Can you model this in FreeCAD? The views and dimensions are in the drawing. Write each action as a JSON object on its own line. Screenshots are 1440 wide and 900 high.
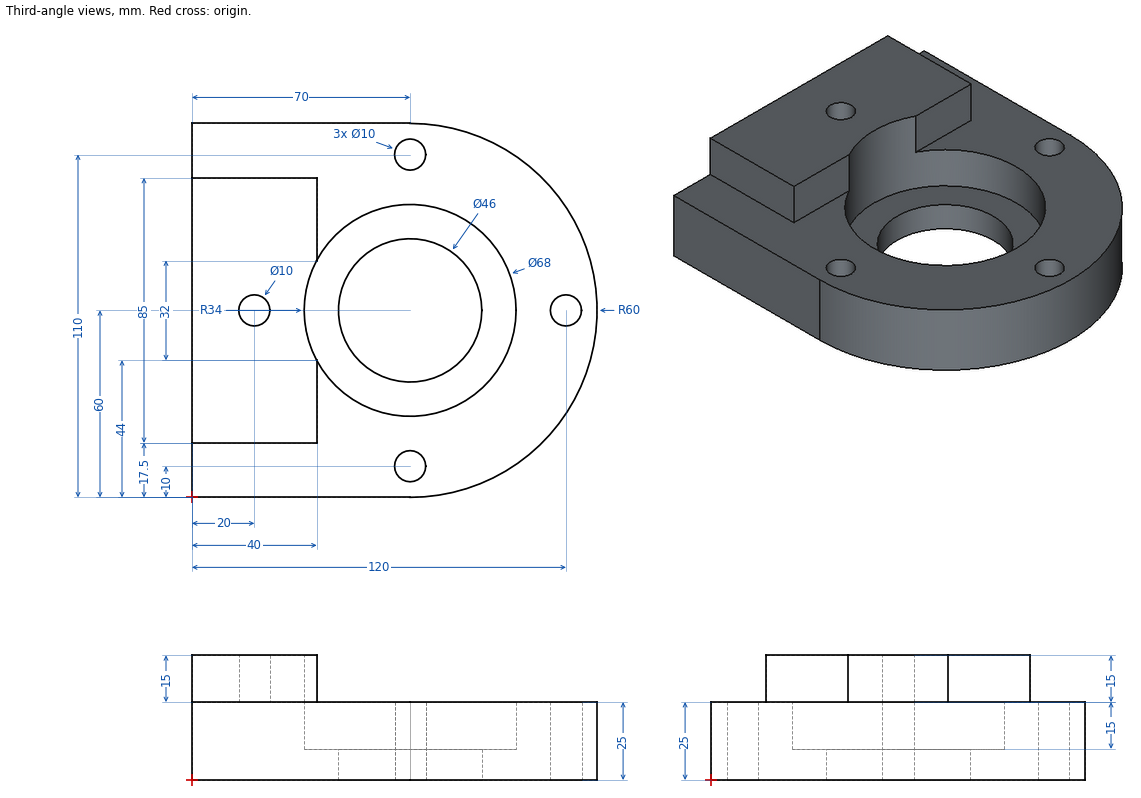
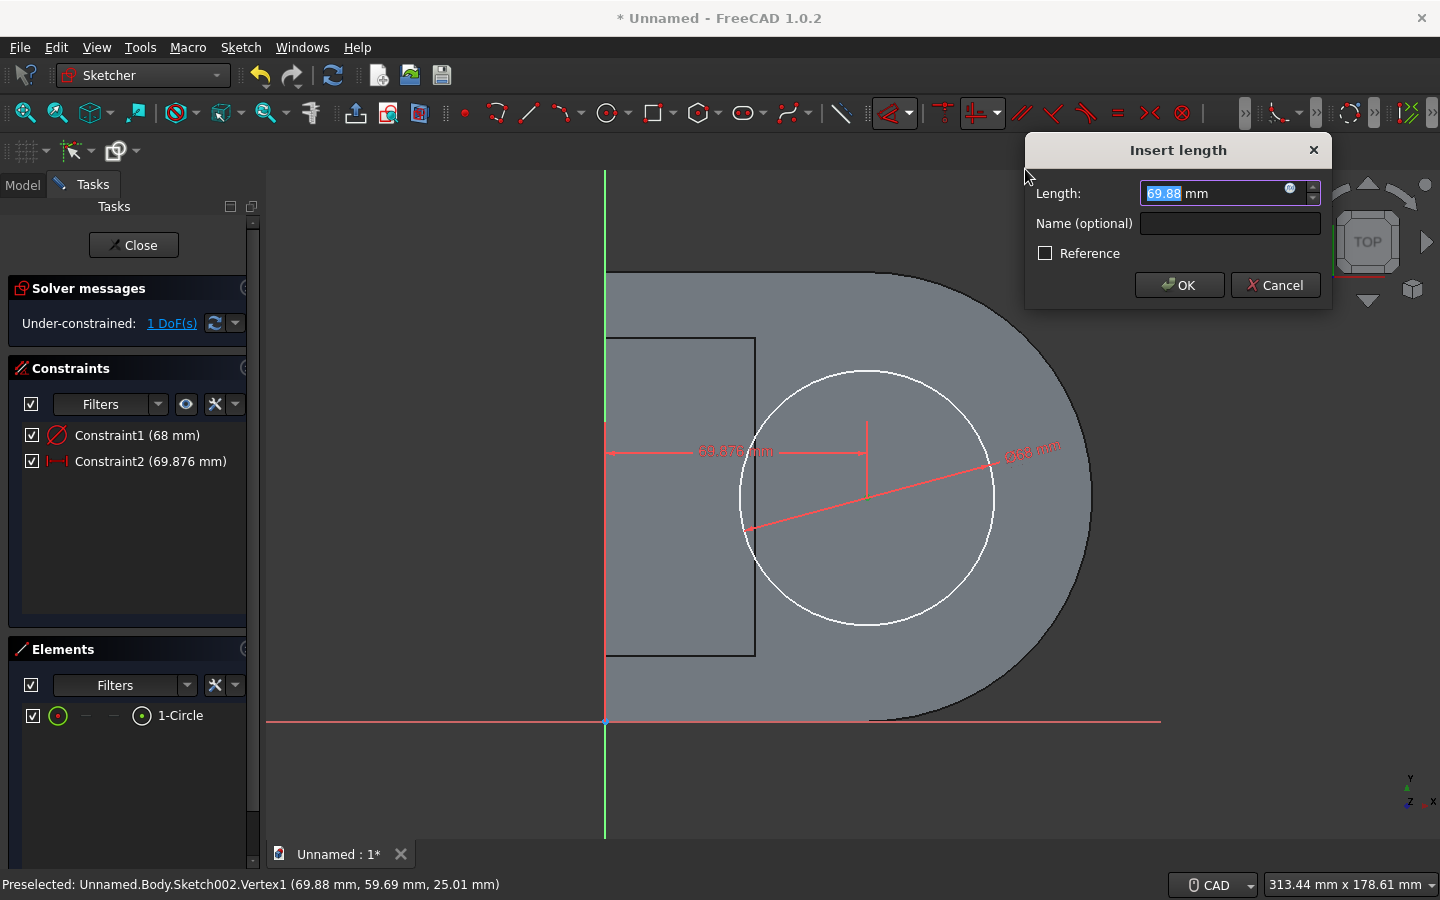
{"action": "type", "text": "70"}
{"action": "key", "text": "Return"}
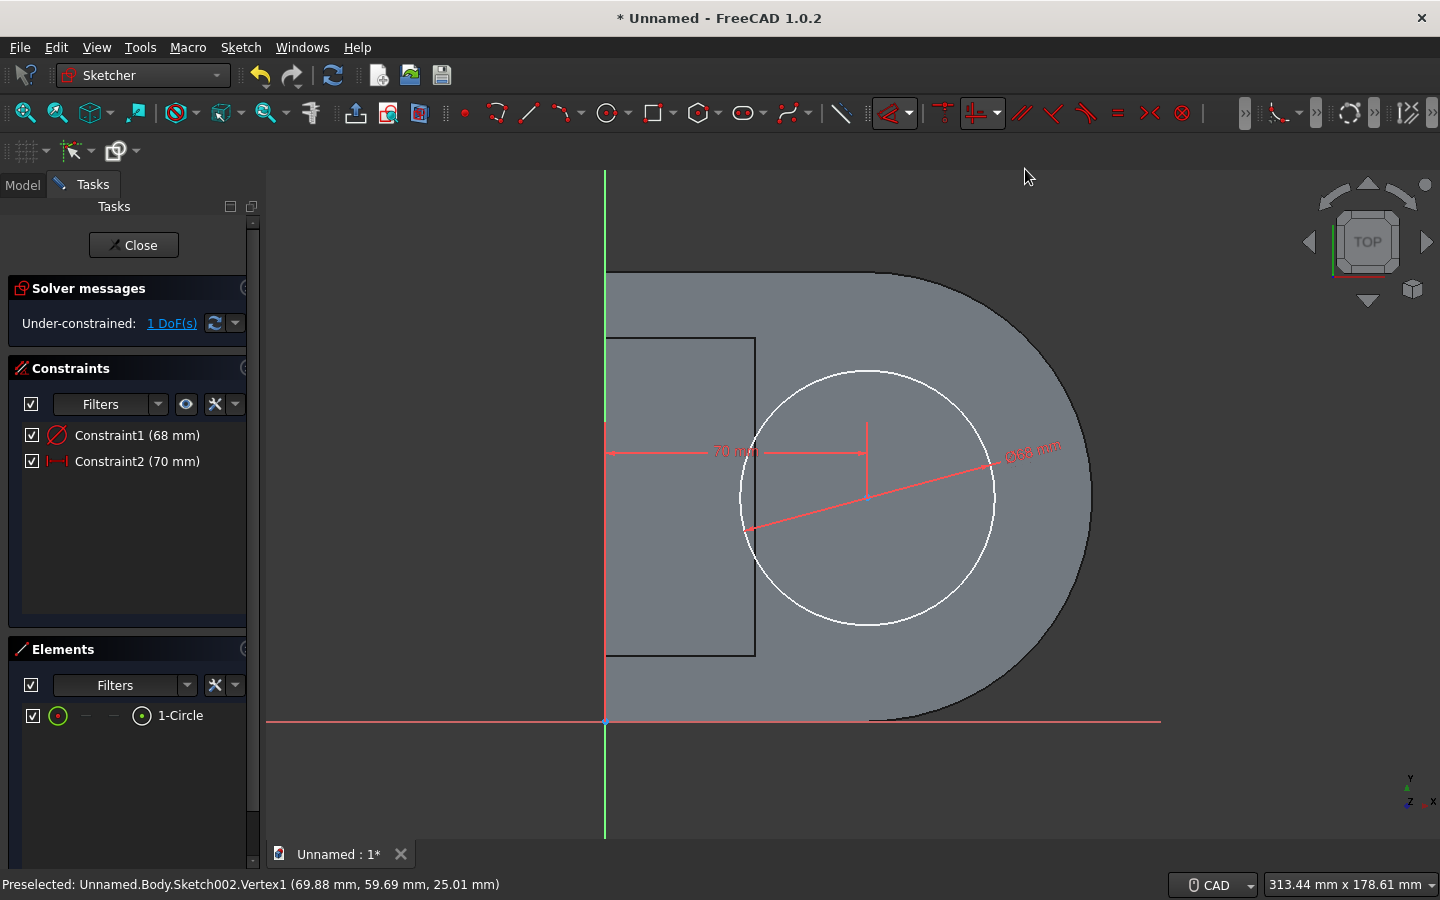
{"action": "left_click", "coordinate": [867, 498]}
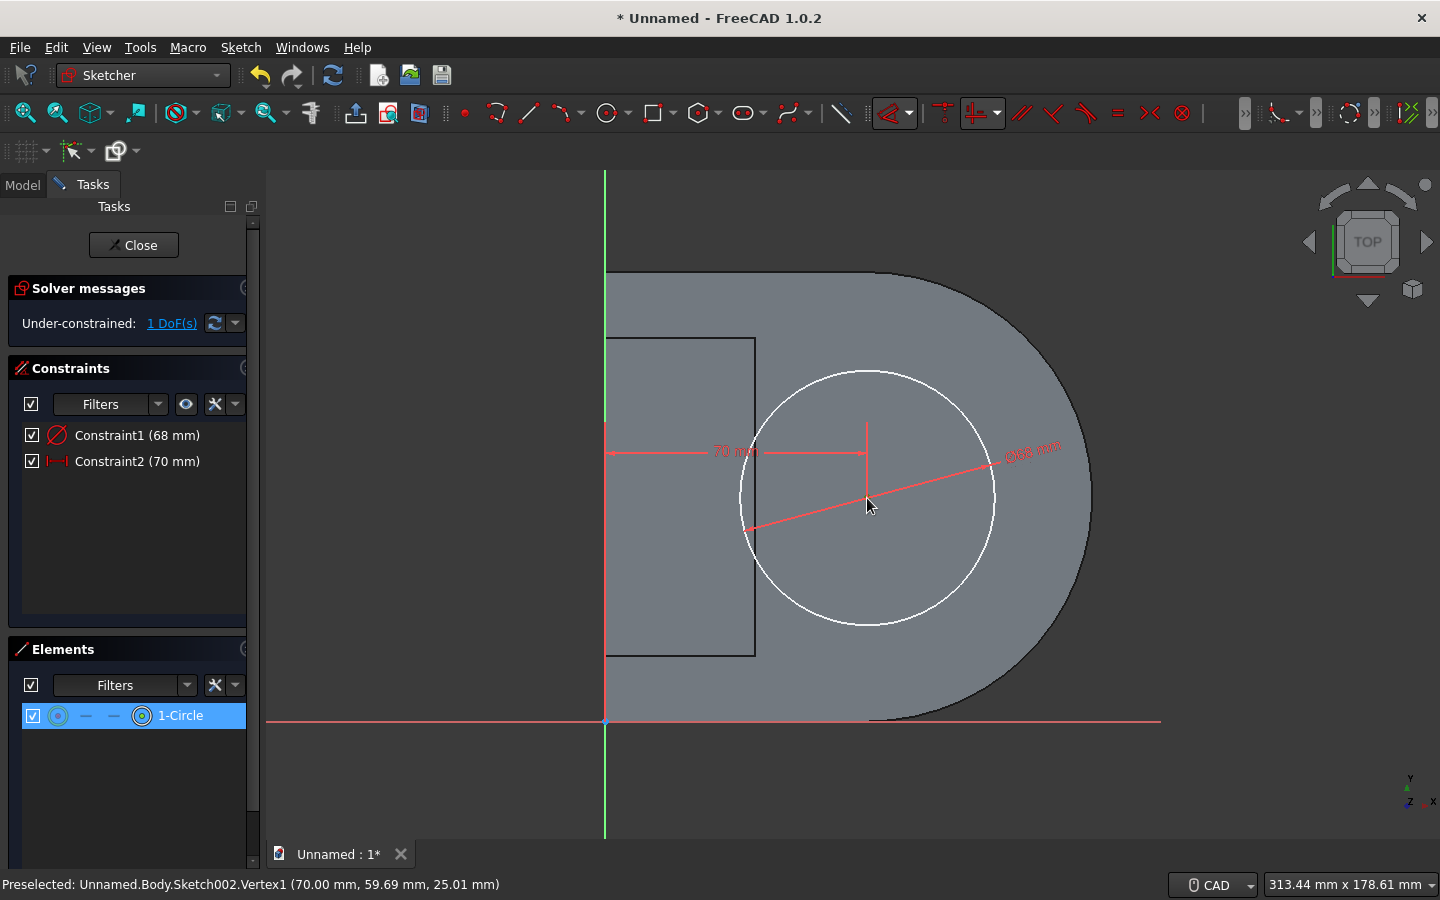
{"action": "left_click", "coordinate": [912, 114]}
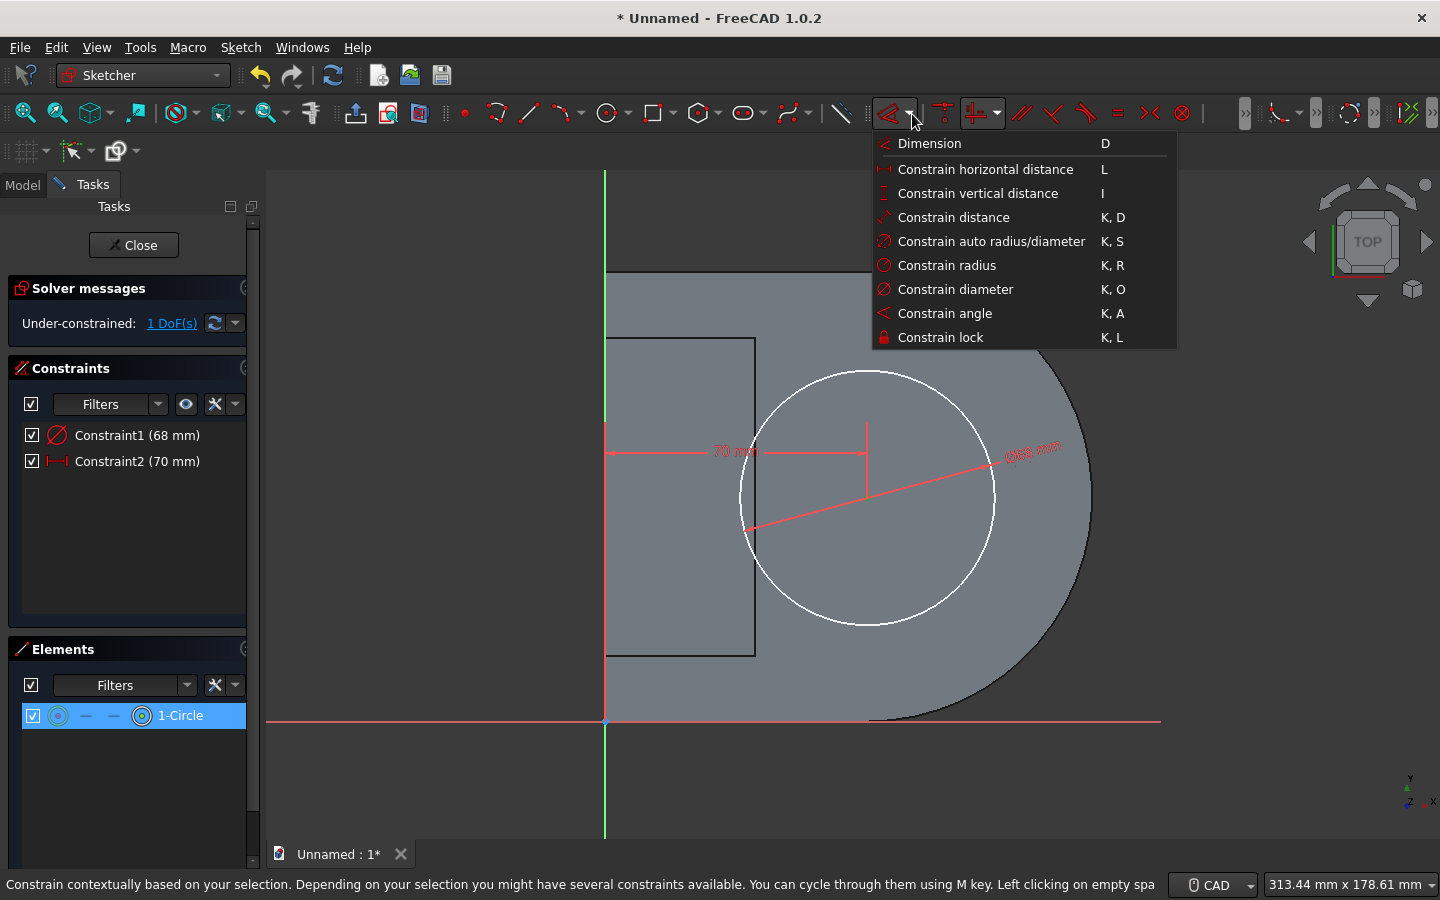
{"action": "left_click", "coordinate": [1025, 193]}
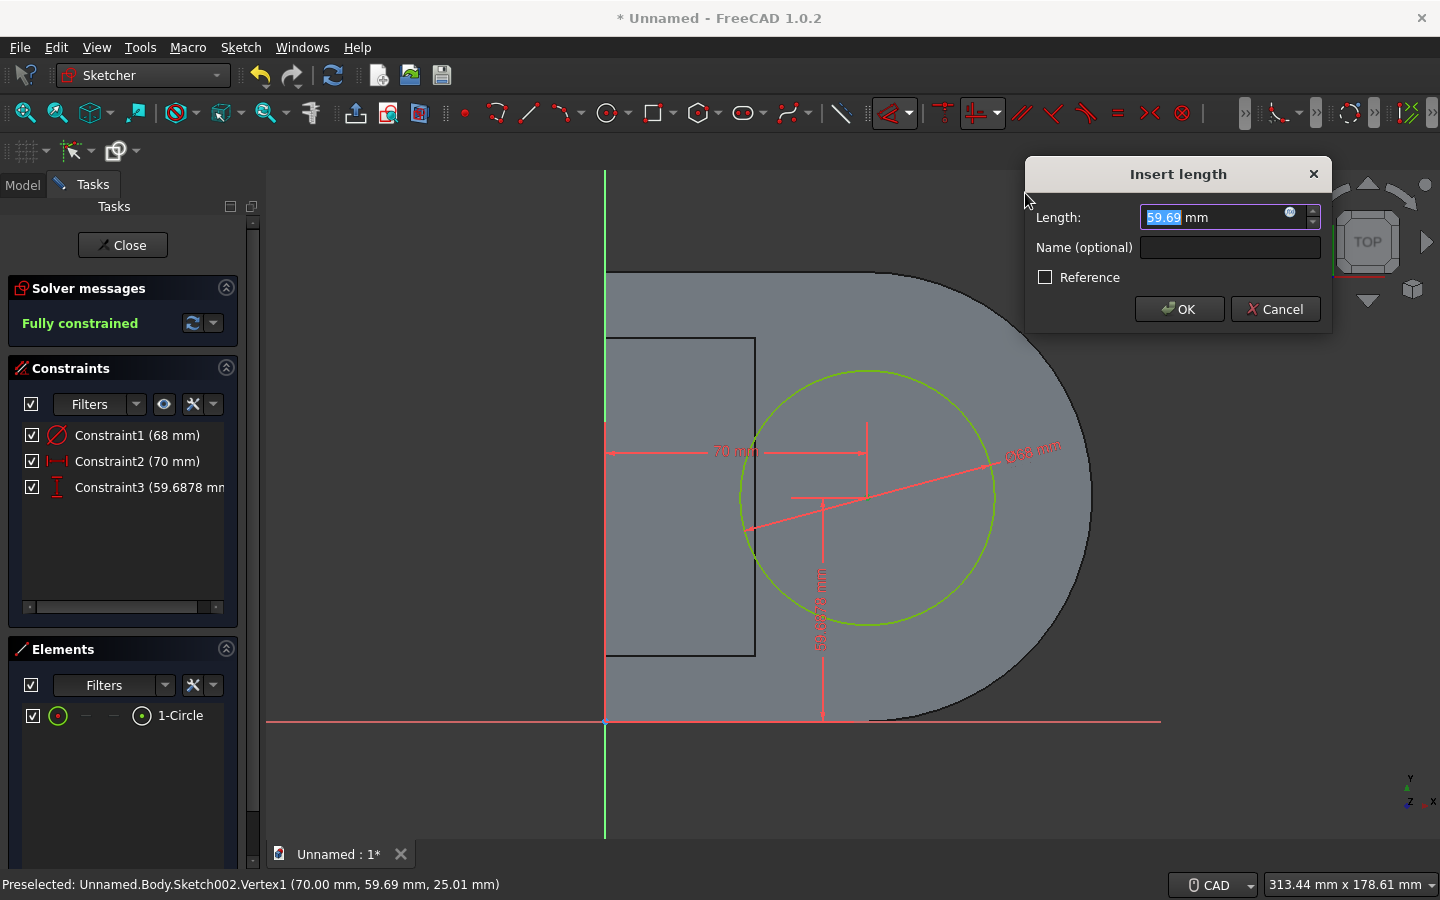
{"action": "type", "text": "60"}
{"action": "key", "text": "Return"}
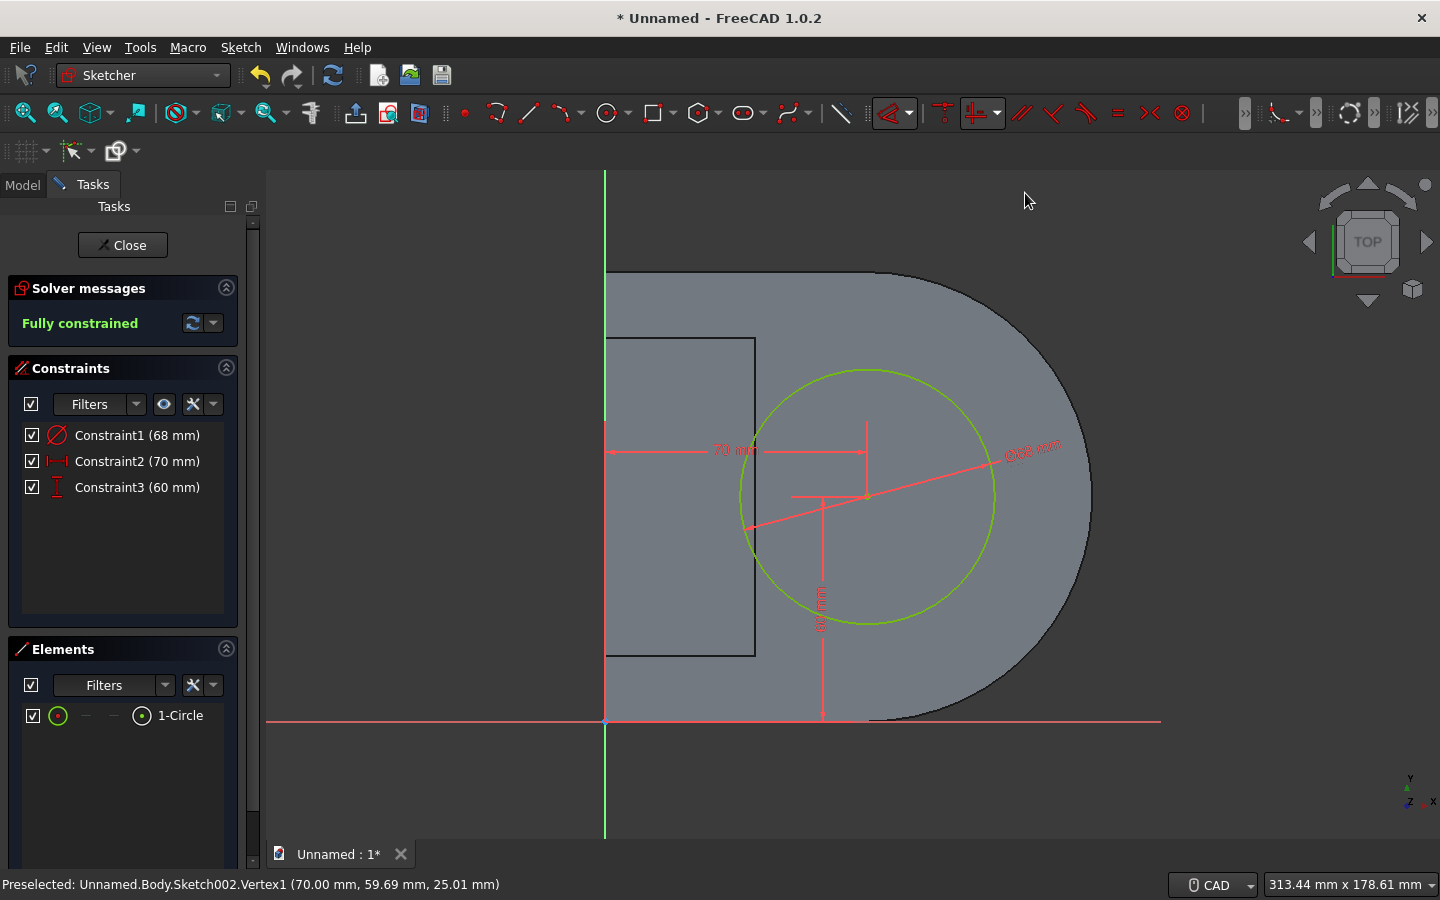
{"action": "left_click", "coordinate": [123, 245]}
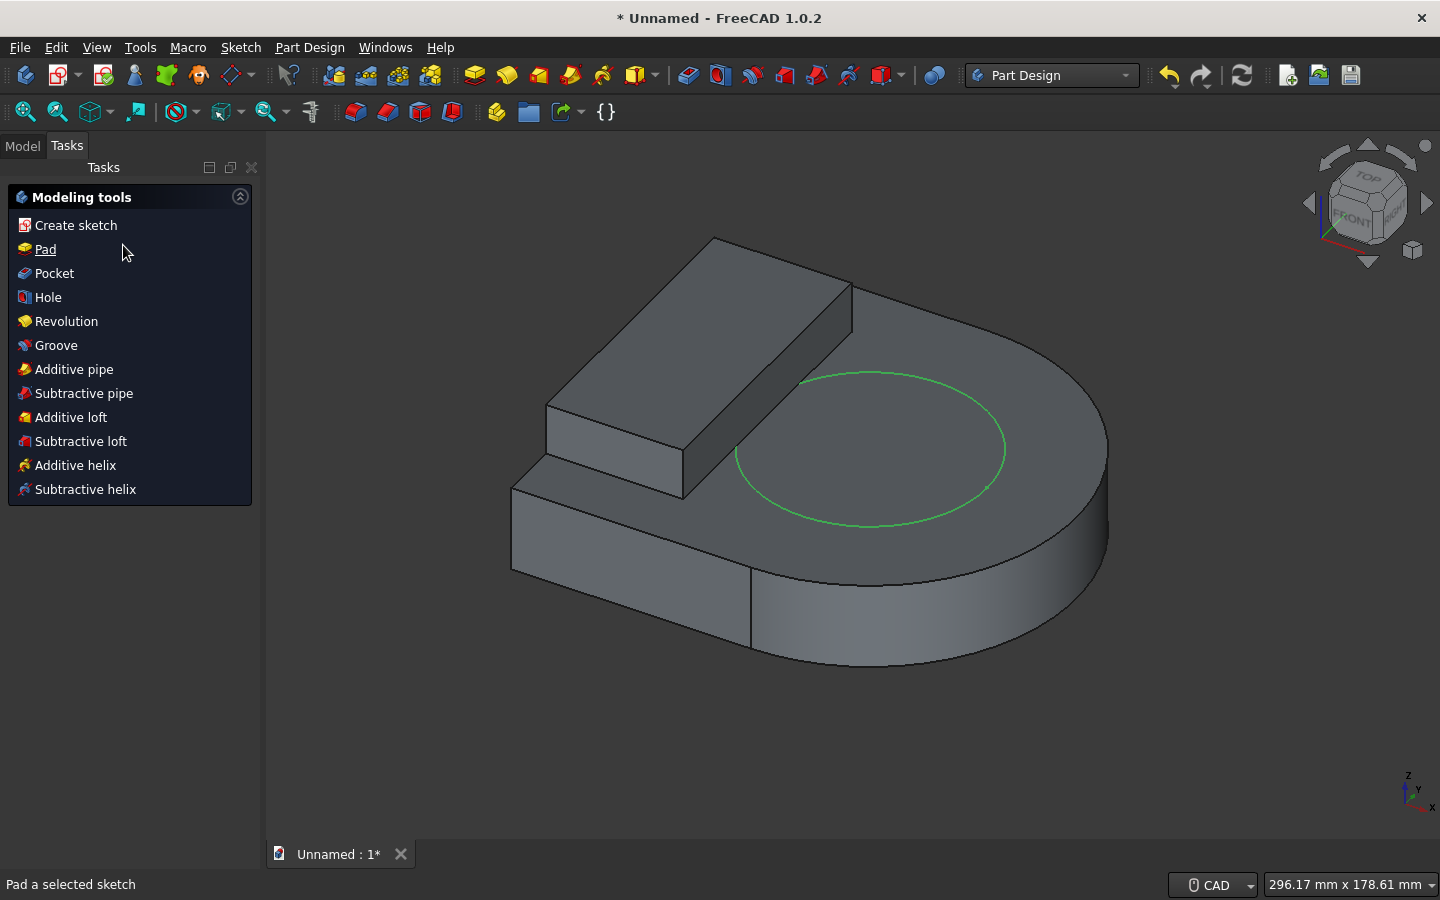
{"action": "left_click", "coordinate": [690, 76]}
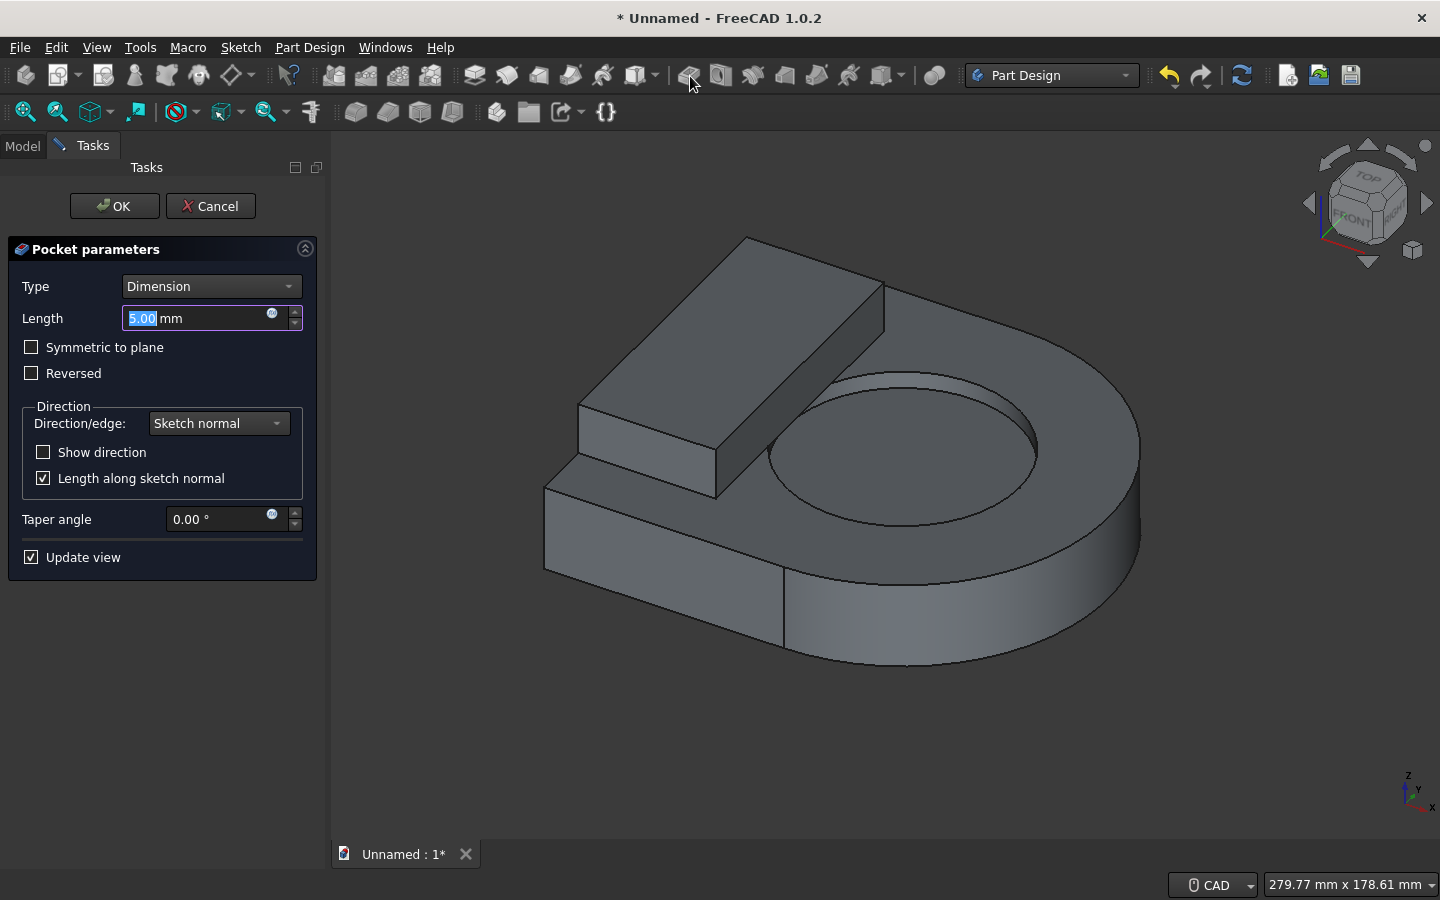
{"action": "type", "text": "15"}
{"action": "key", "text": "Tab"}